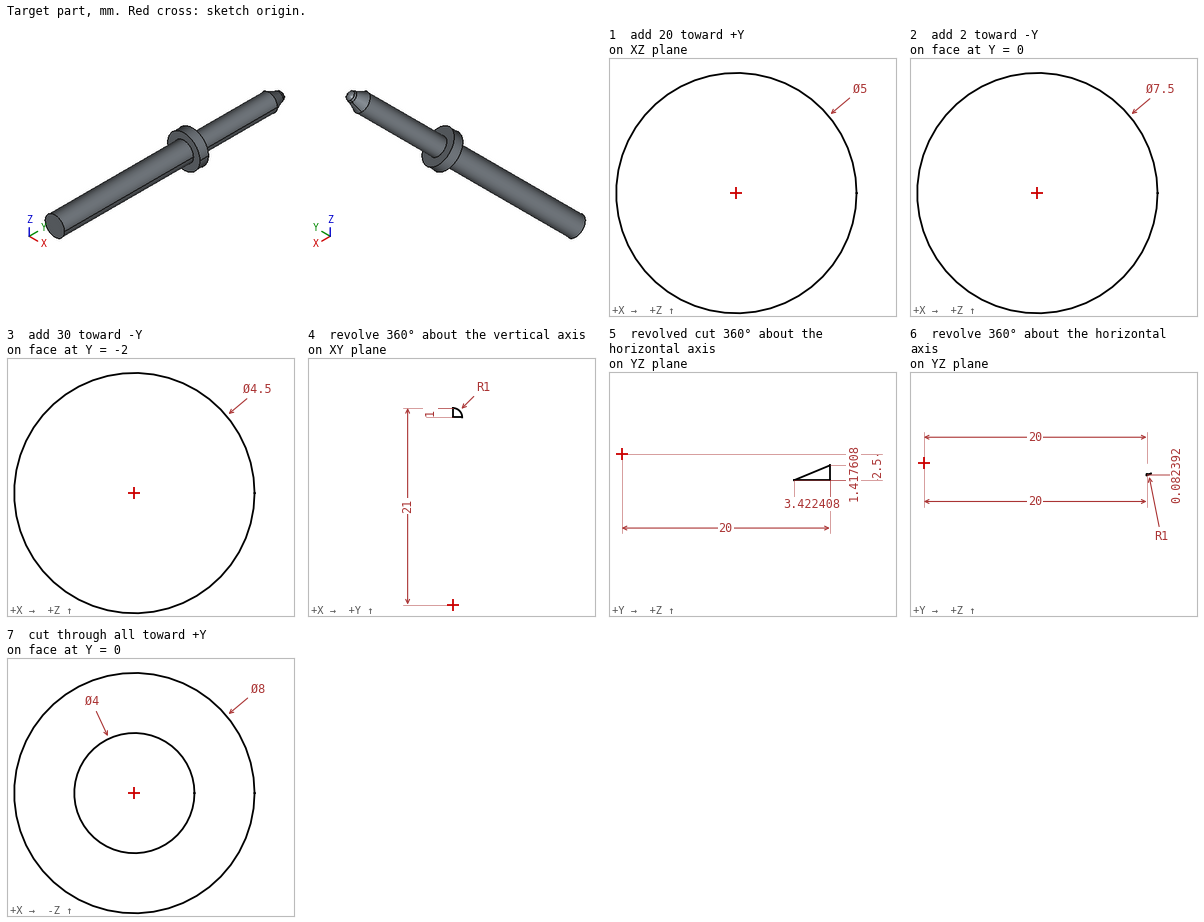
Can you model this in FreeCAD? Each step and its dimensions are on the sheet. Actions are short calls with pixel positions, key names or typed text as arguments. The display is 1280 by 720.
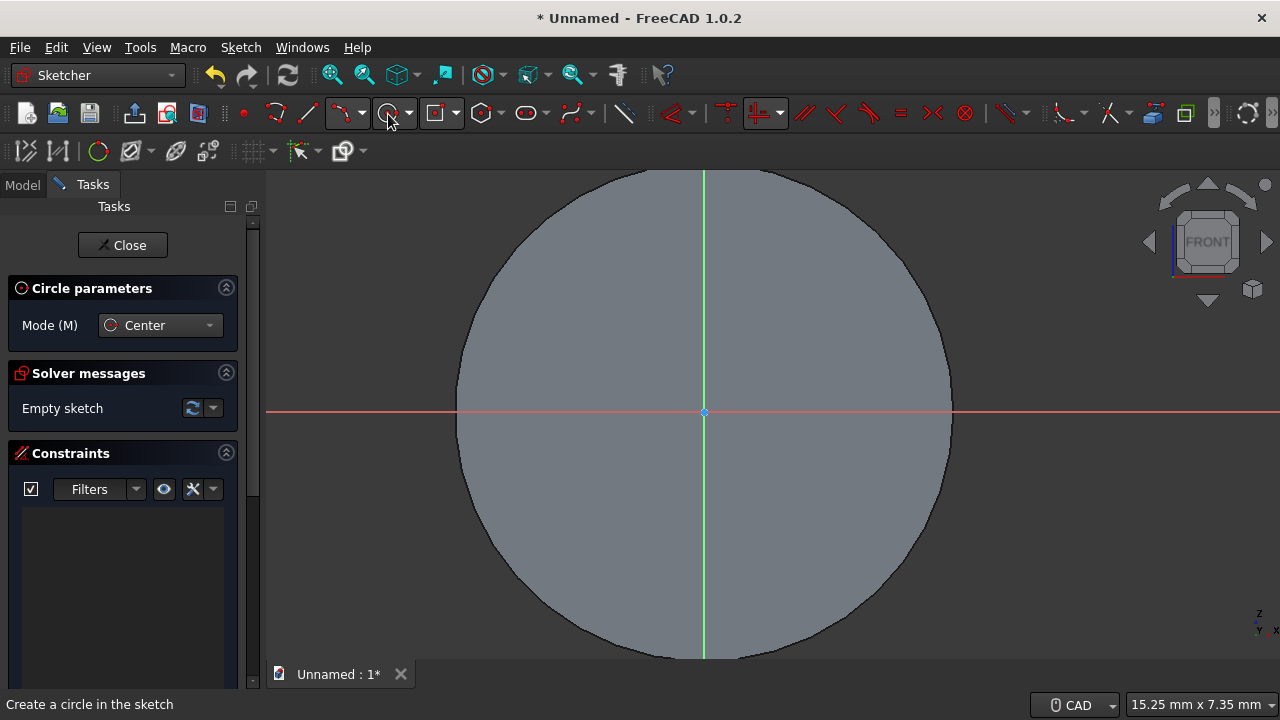
click(704, 412)
click(810, 306)
key(Escape)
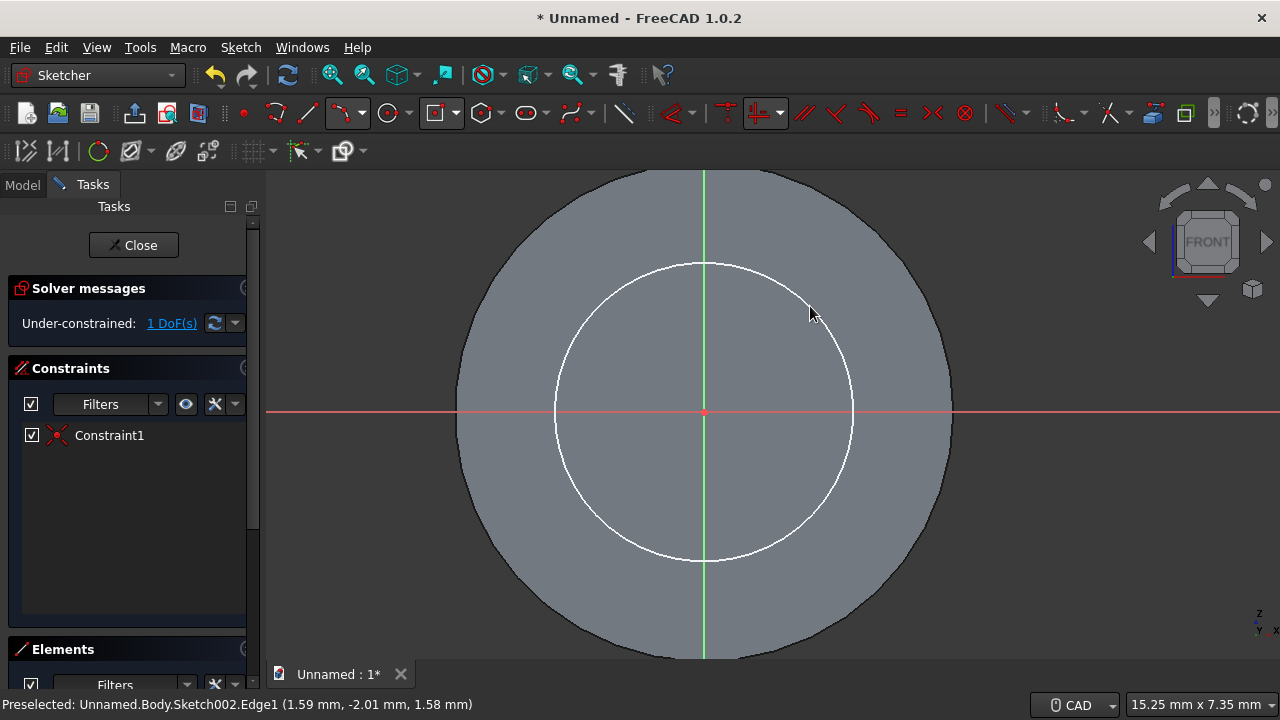
click(672, 114)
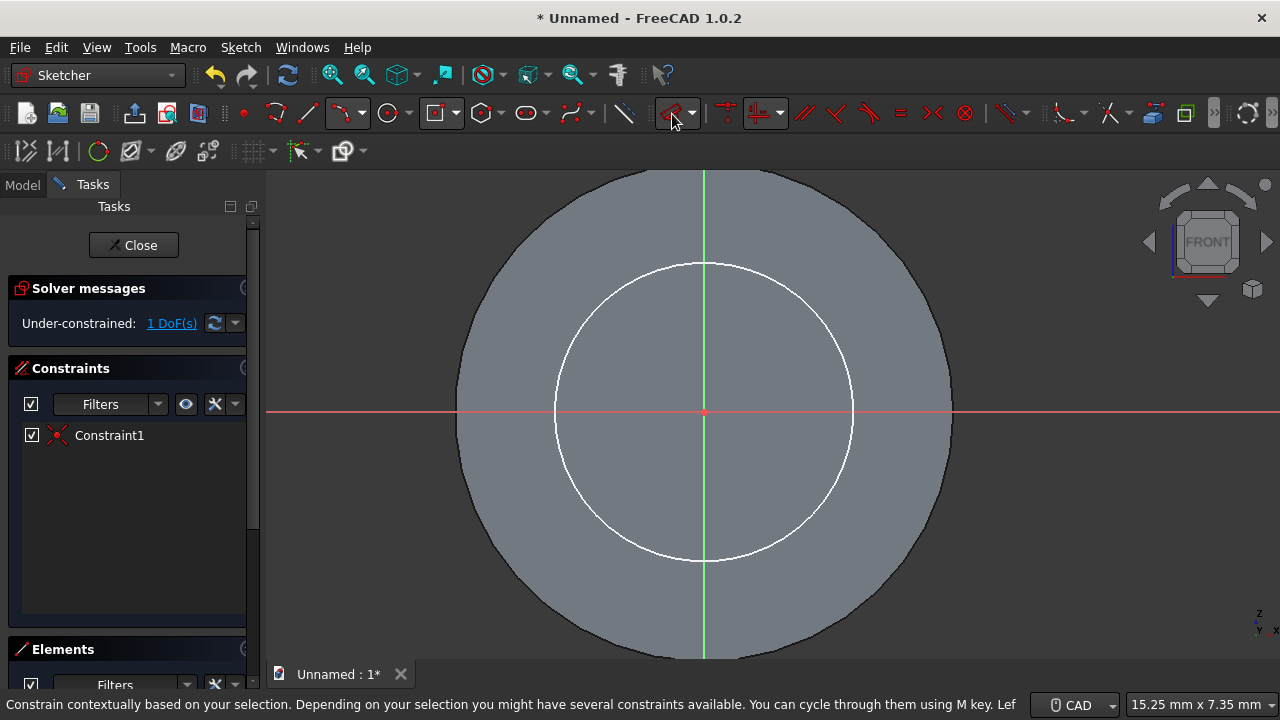
click(809, 306)
click(831, 283)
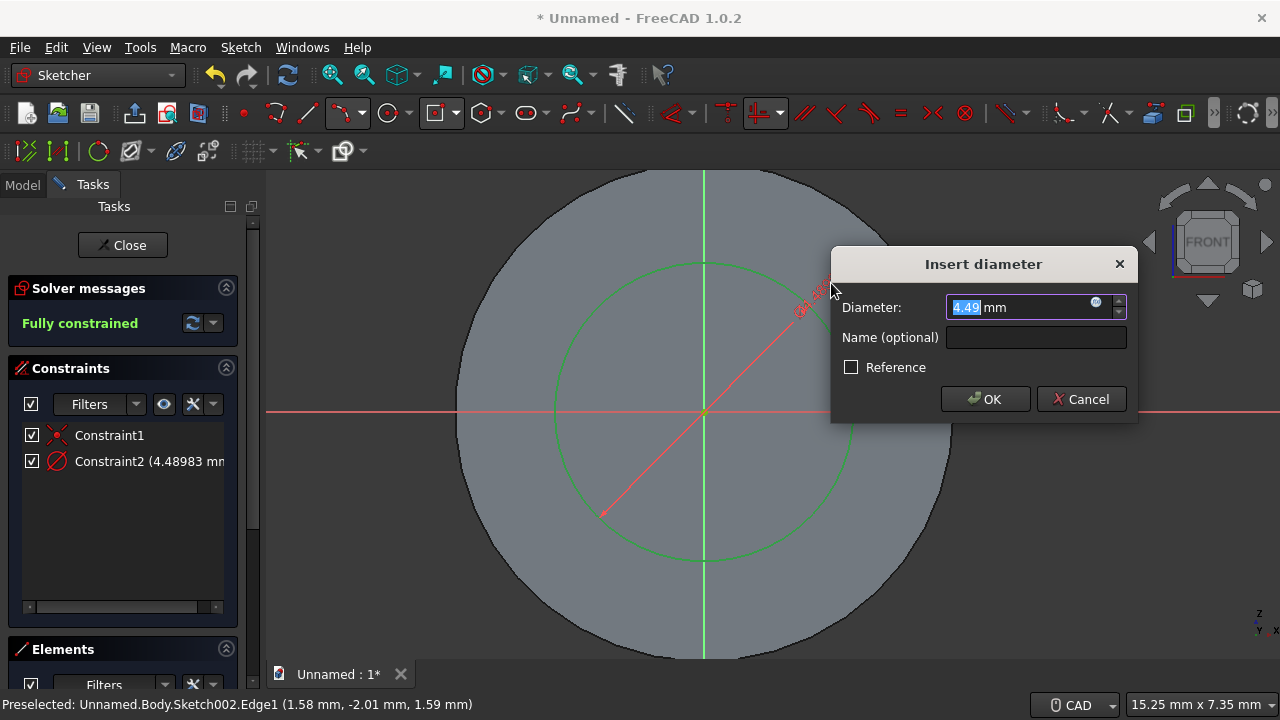
text(4.5)
key(Return)
key(Escape)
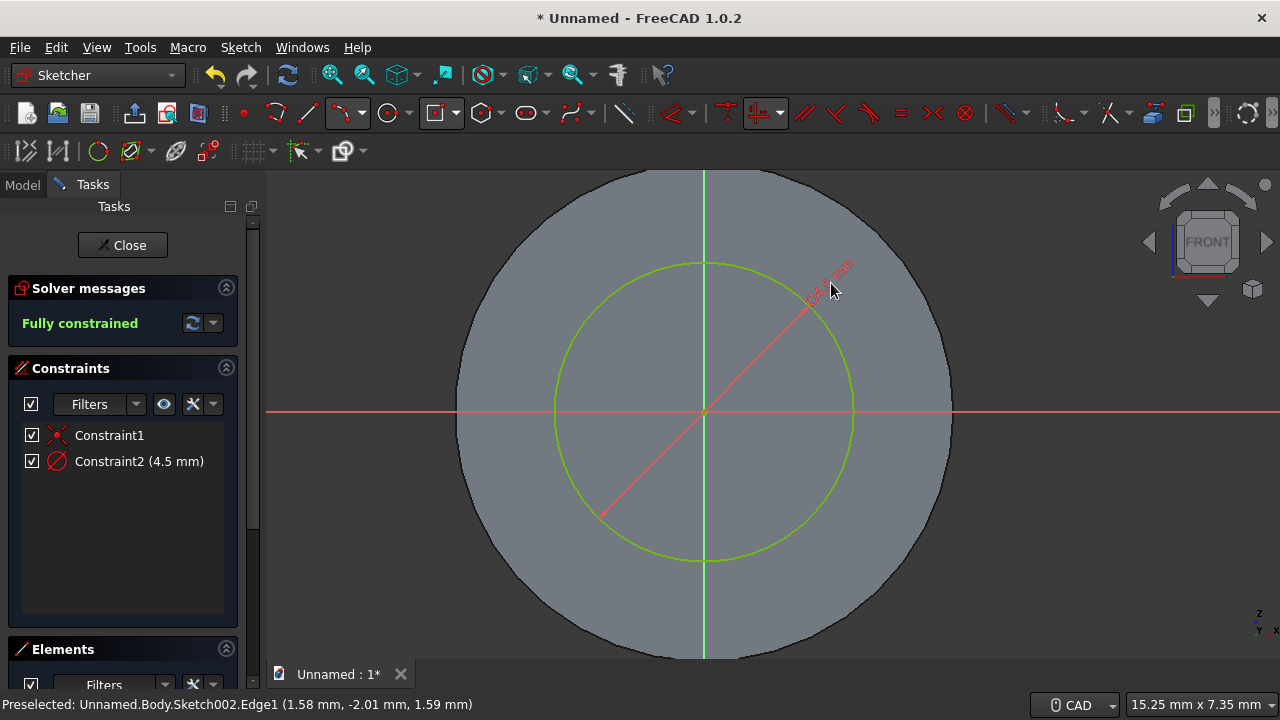
click(123, 245)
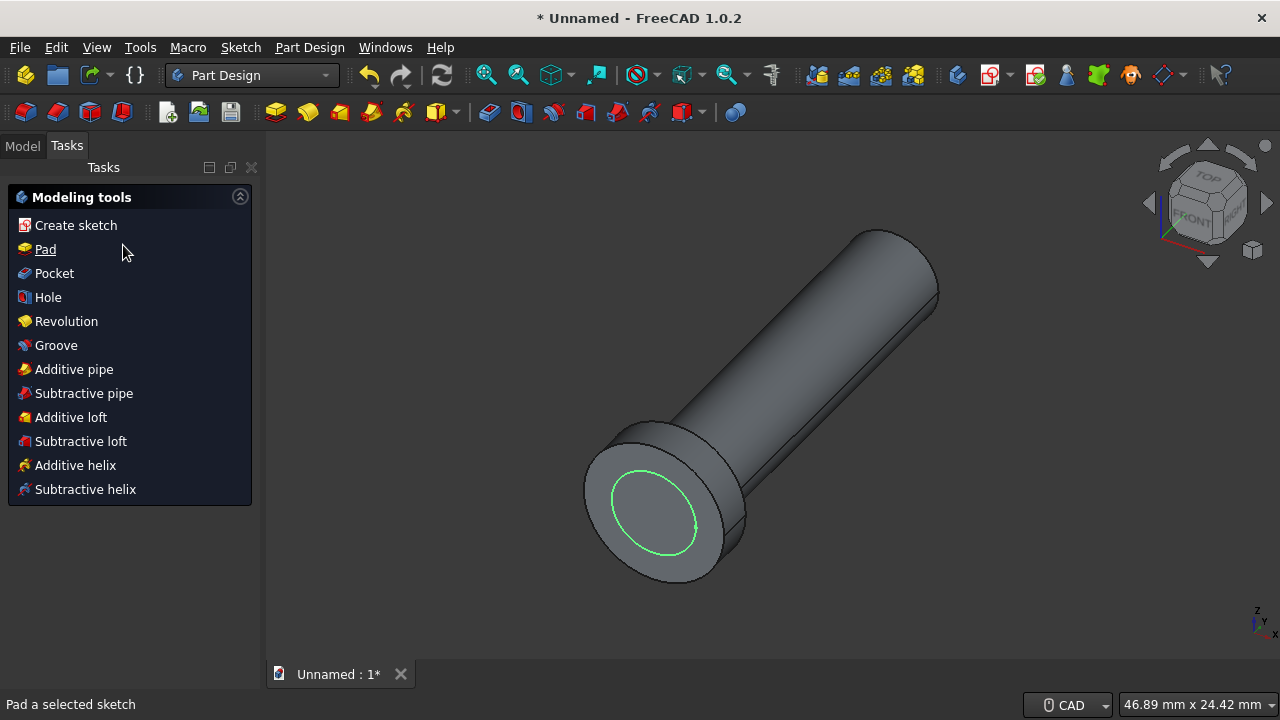
click(276, 112)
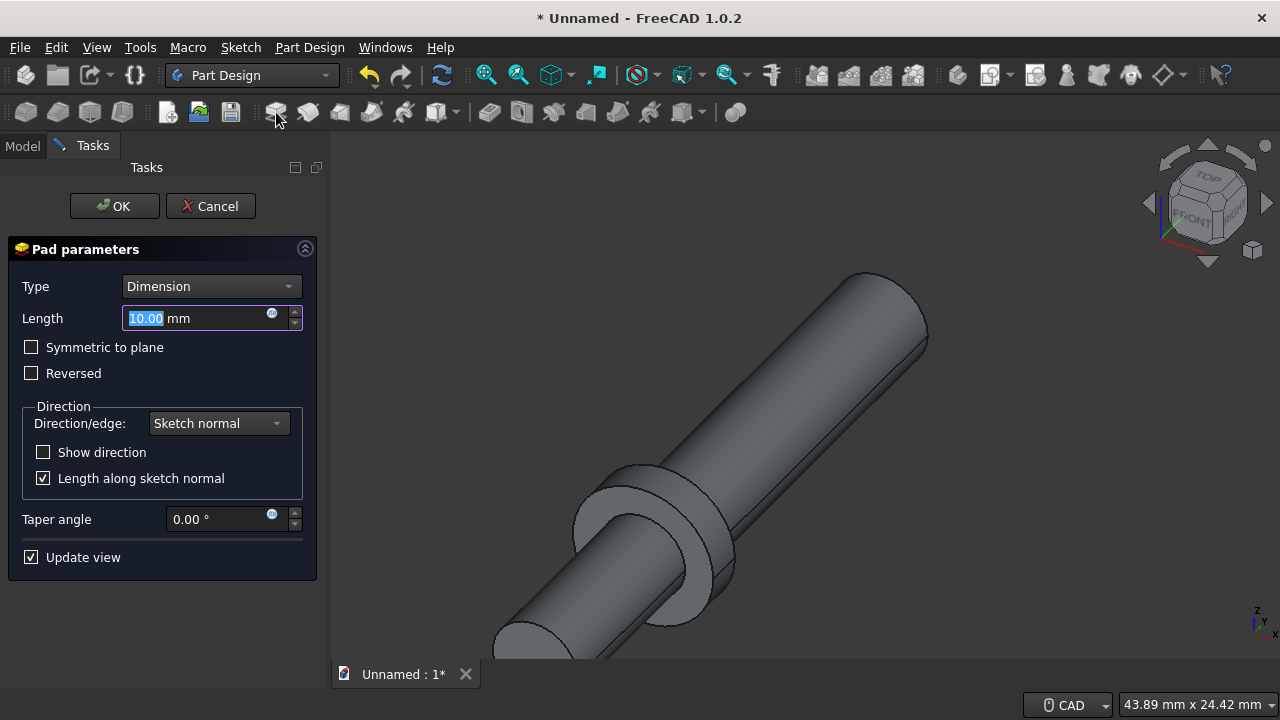
text(30)
key(Tab)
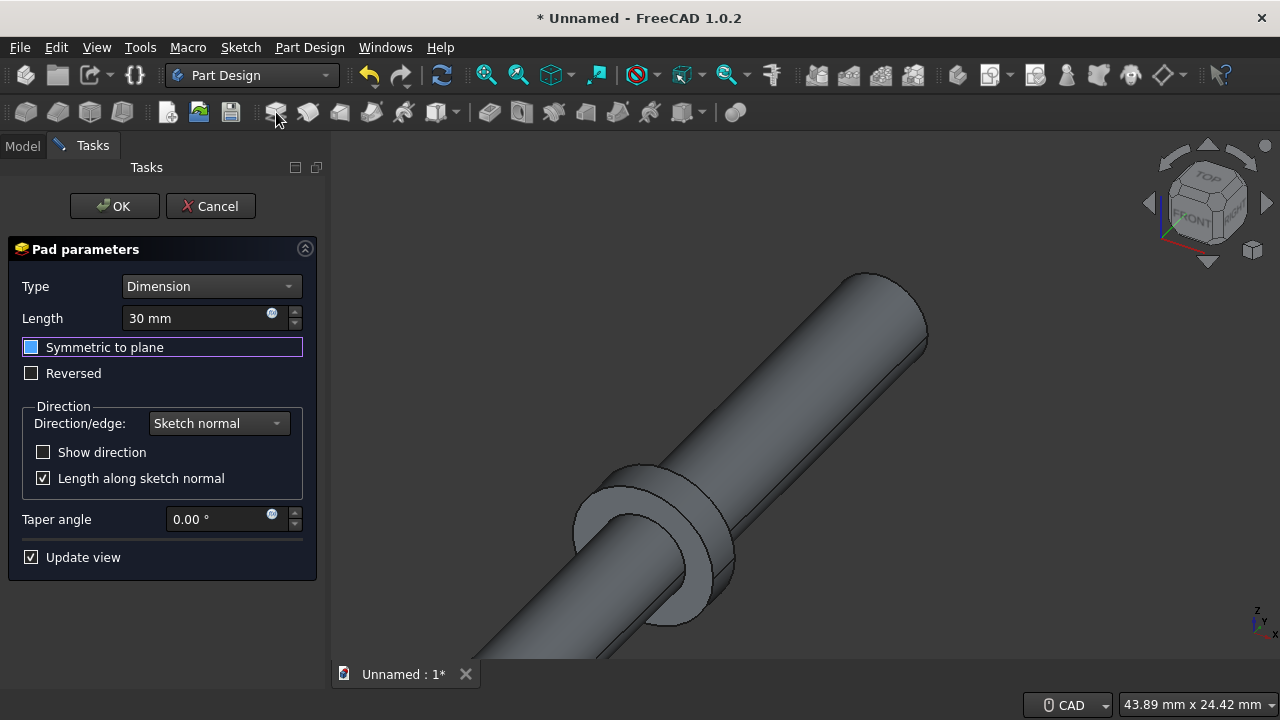
click(115, 206)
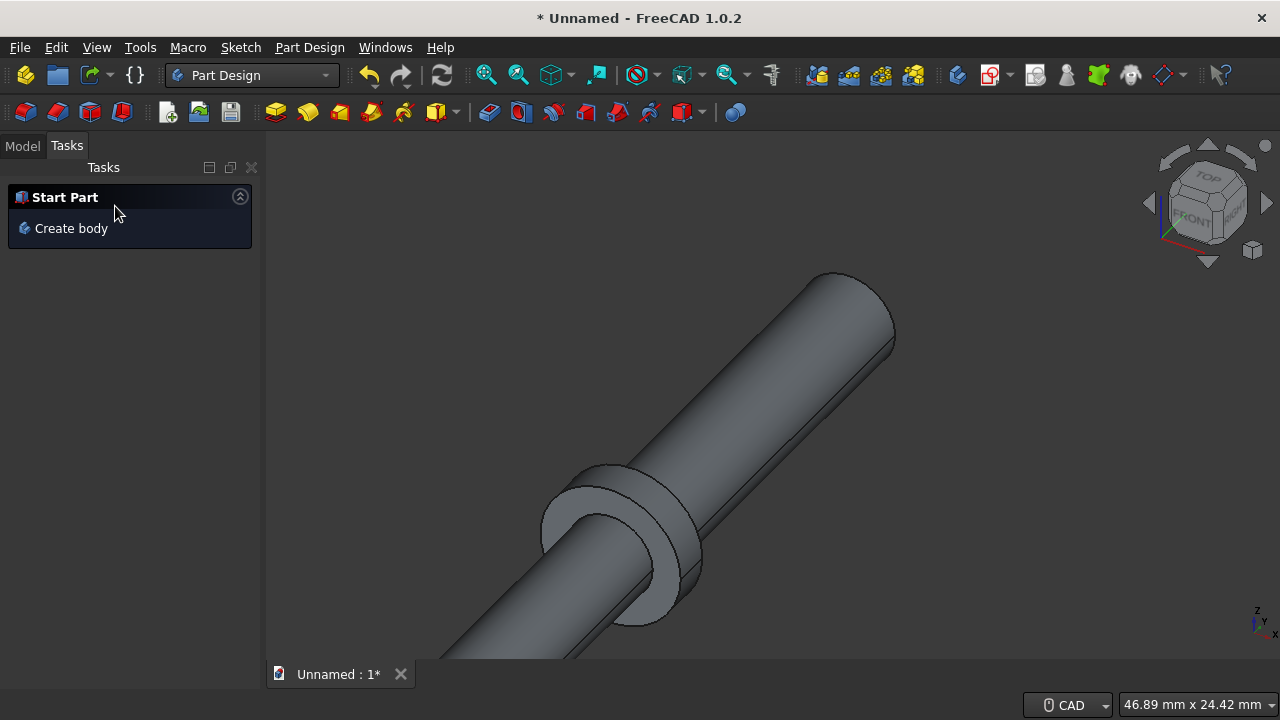
click(488, 76)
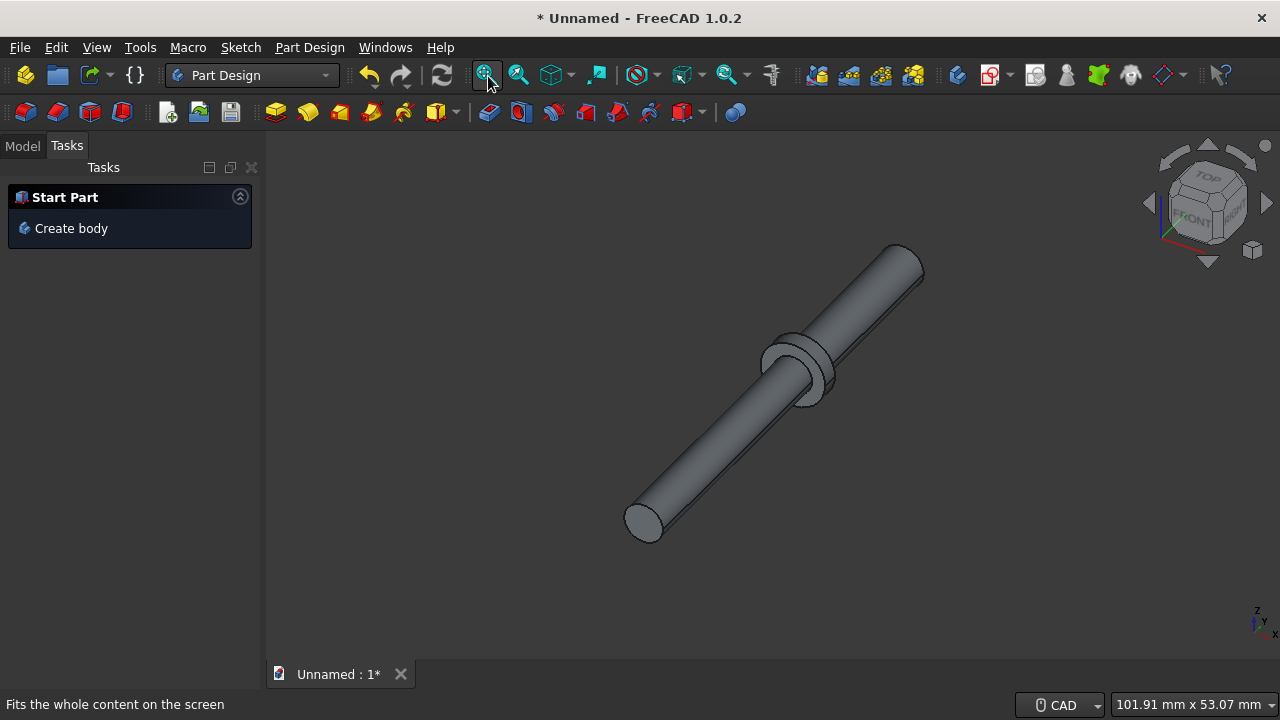
click(990, 76)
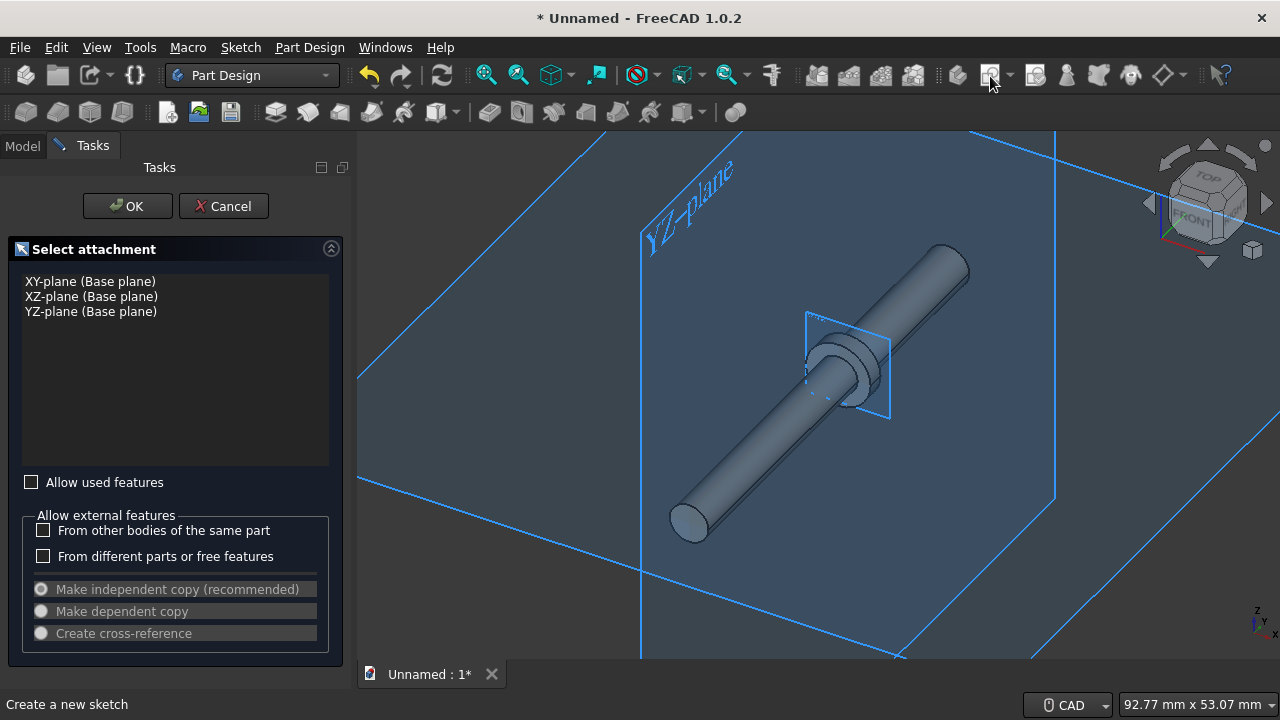
click(82, 282)